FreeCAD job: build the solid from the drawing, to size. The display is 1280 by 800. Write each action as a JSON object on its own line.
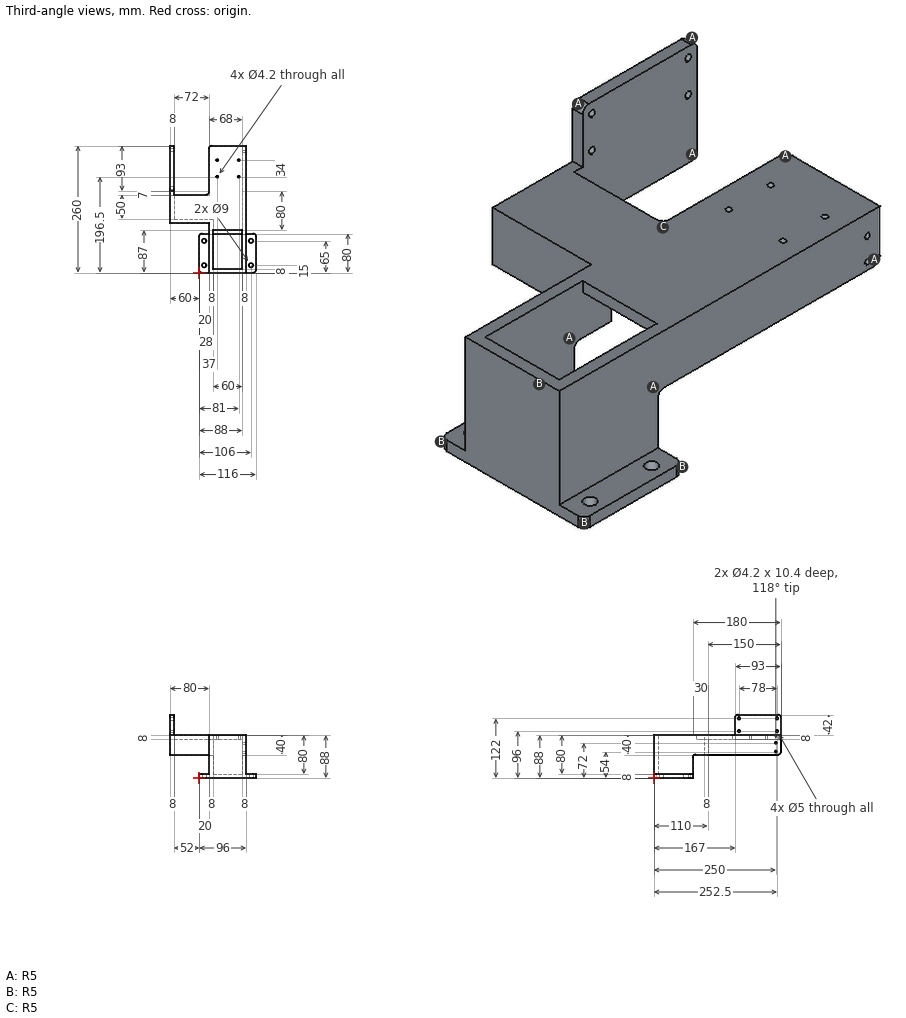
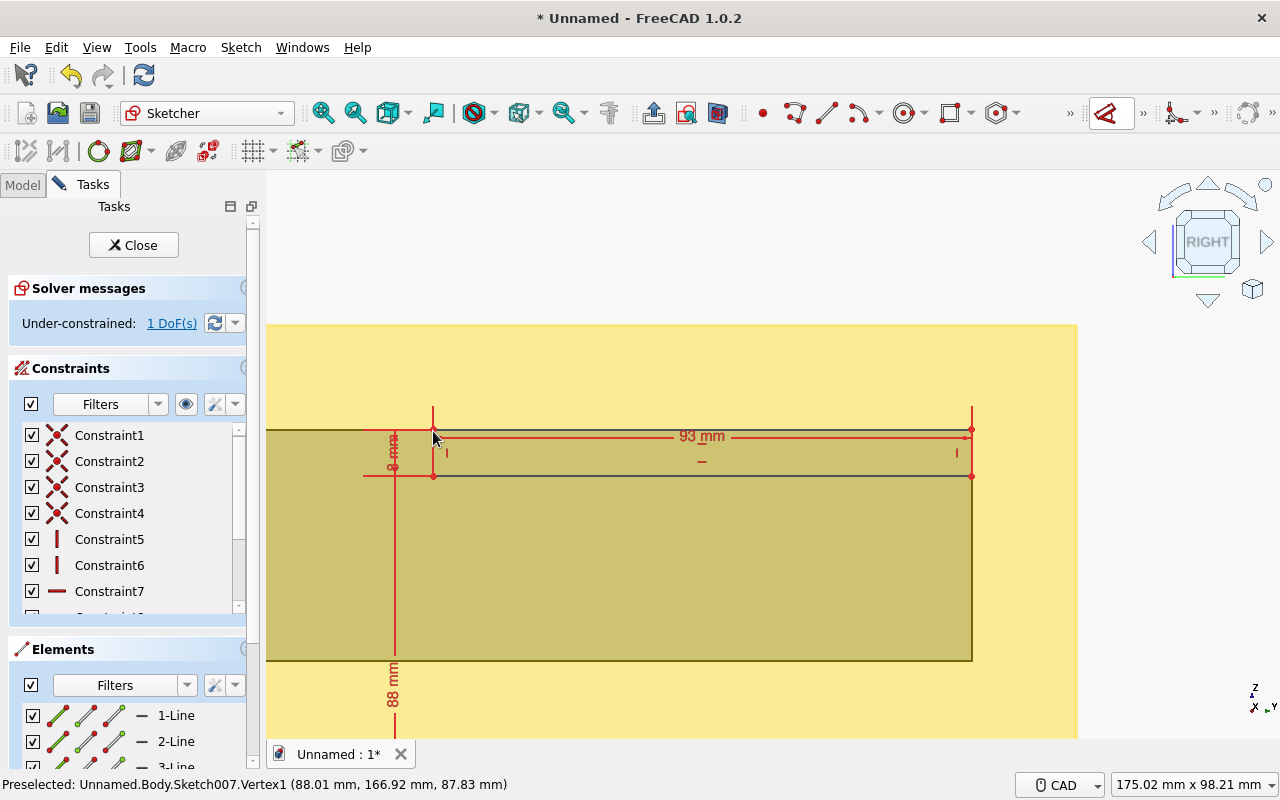
{"action": "left_click", "coordinate": [433, 430]}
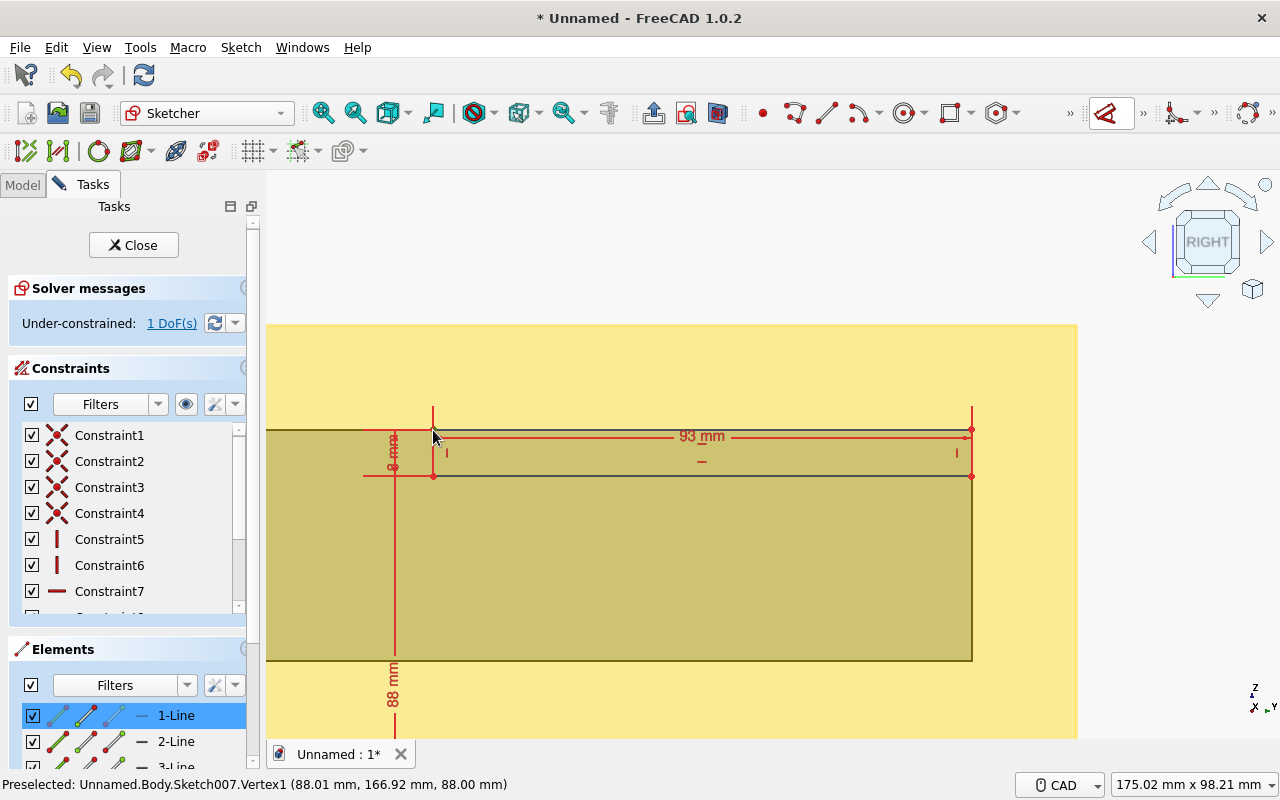
{"action": "key", "text": "l"}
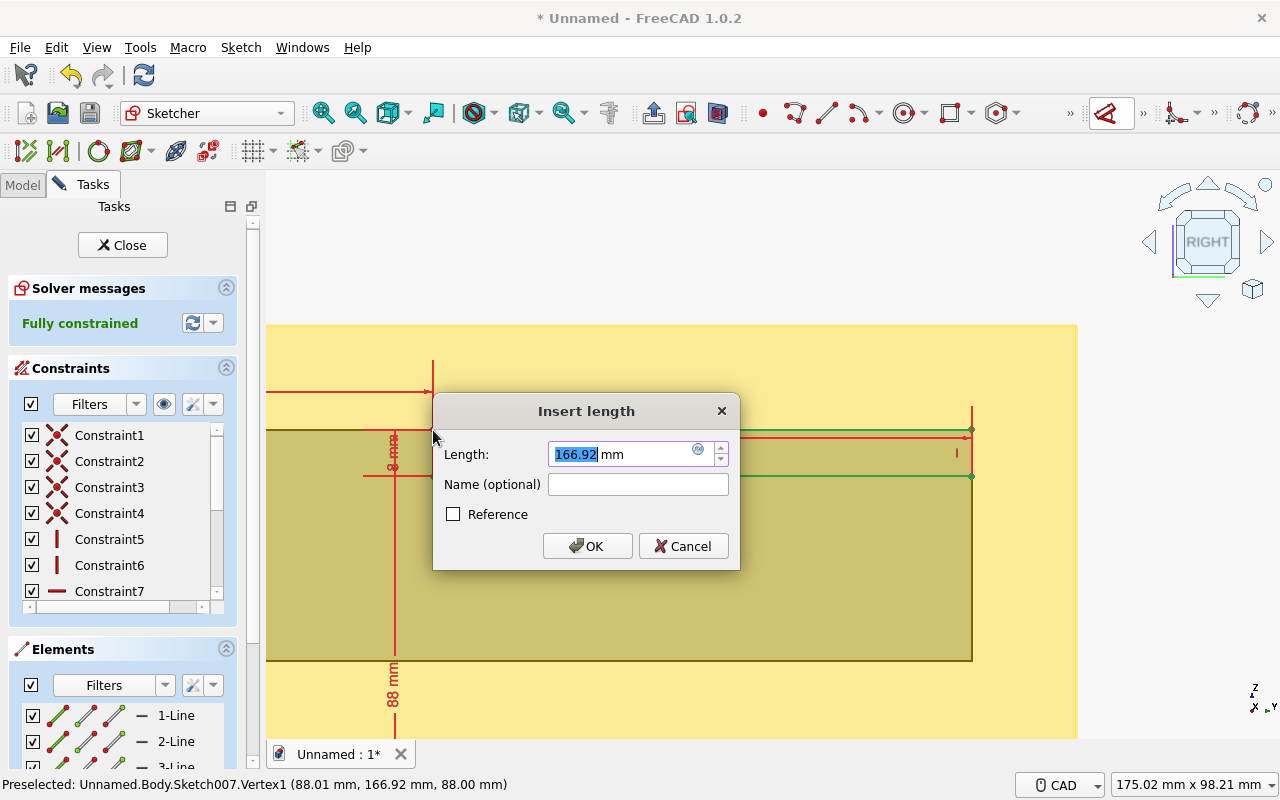
{"action": "type", "text": "167"}
{"action": "key", "text": "Return"}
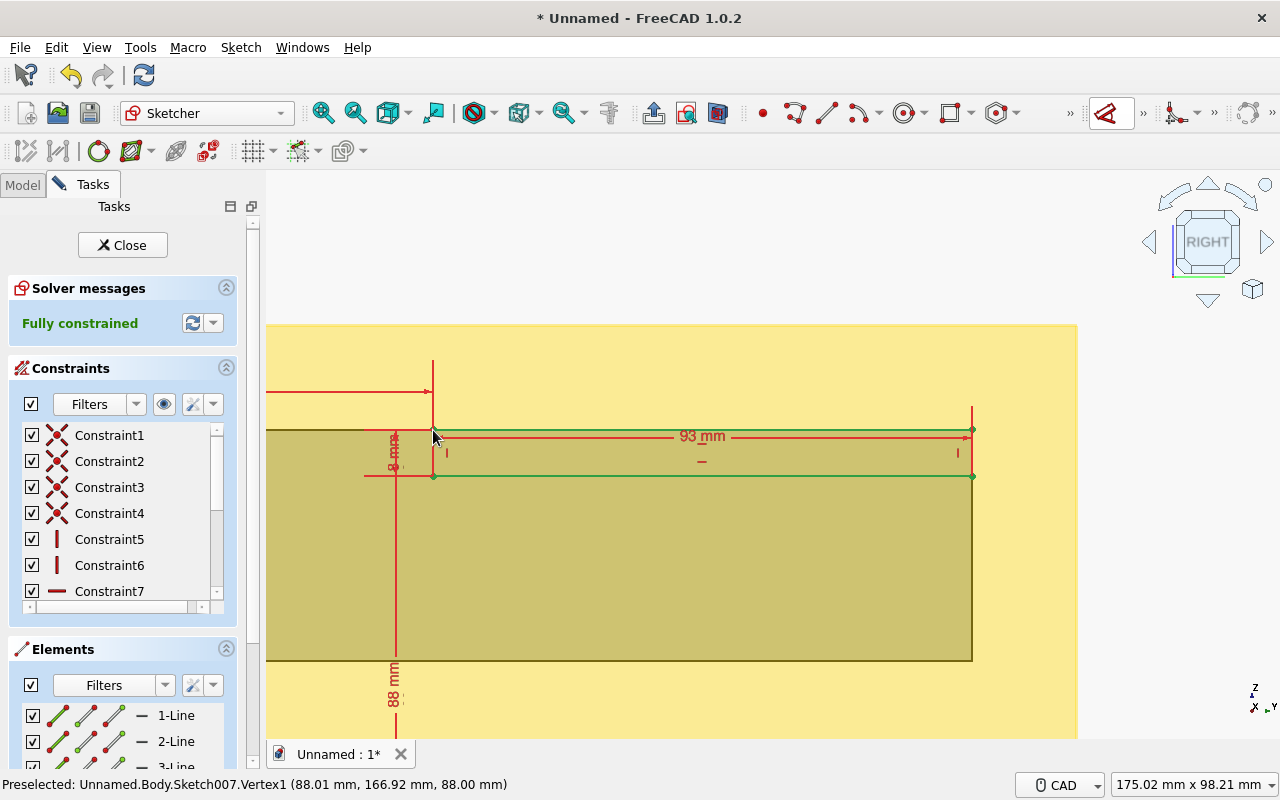
{"action": "left_click", "coordinate": [123, 245]}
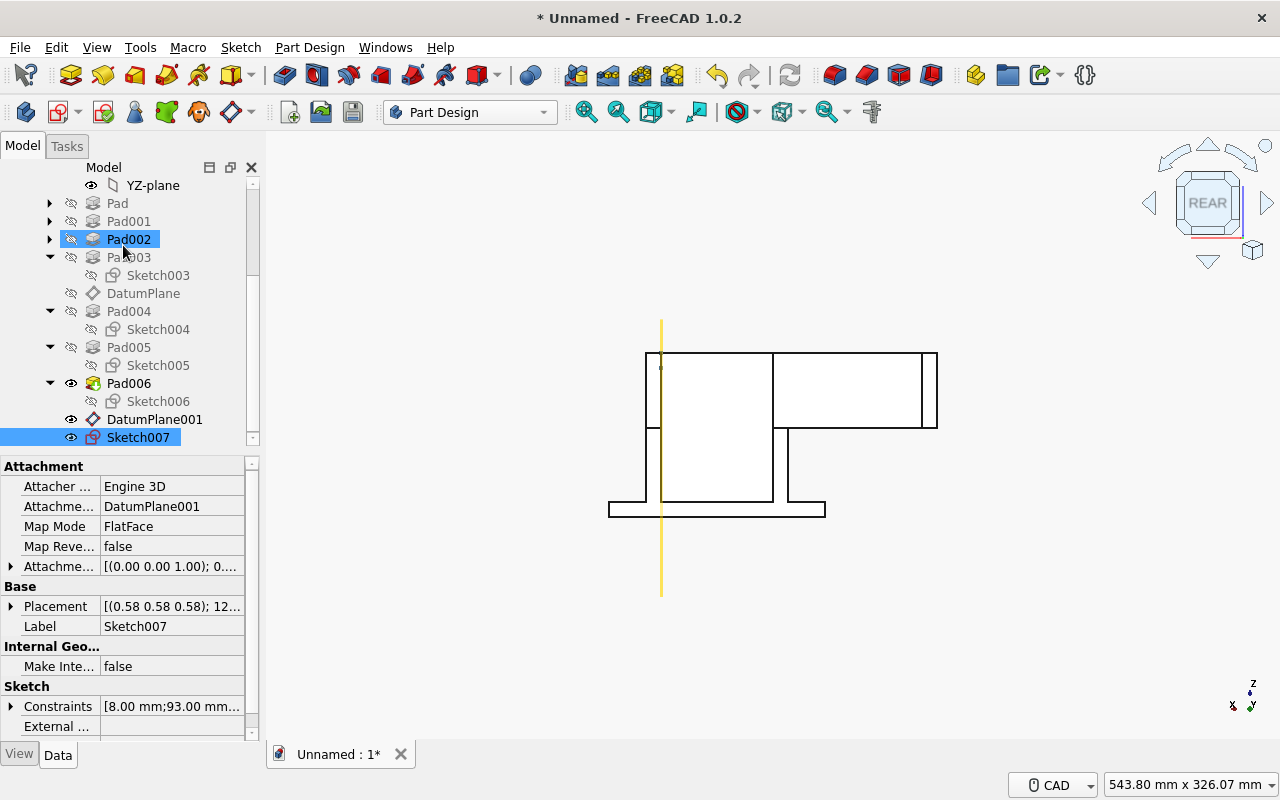
{"action": "left_click", "coordinate": [72, 76]}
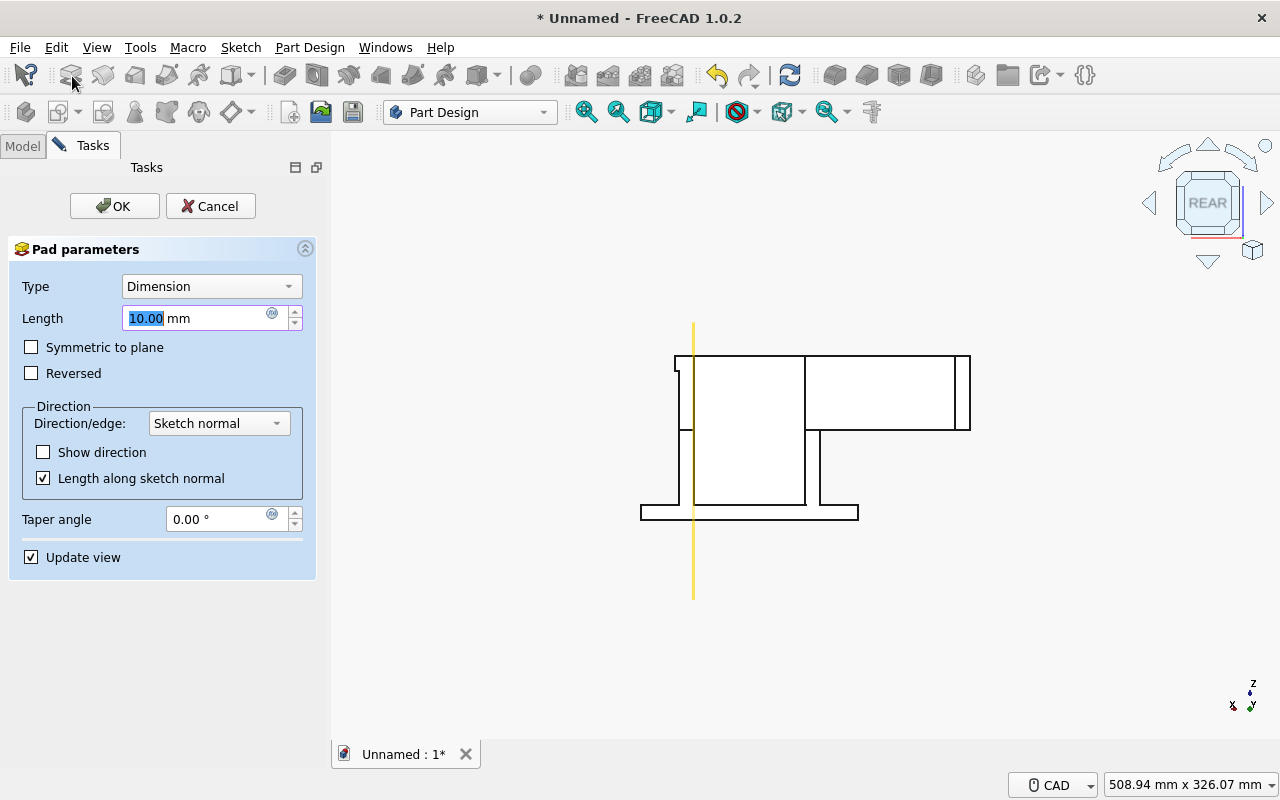
{"action": "type", "text": "68"}
{"action": "key", "text": "Tab"}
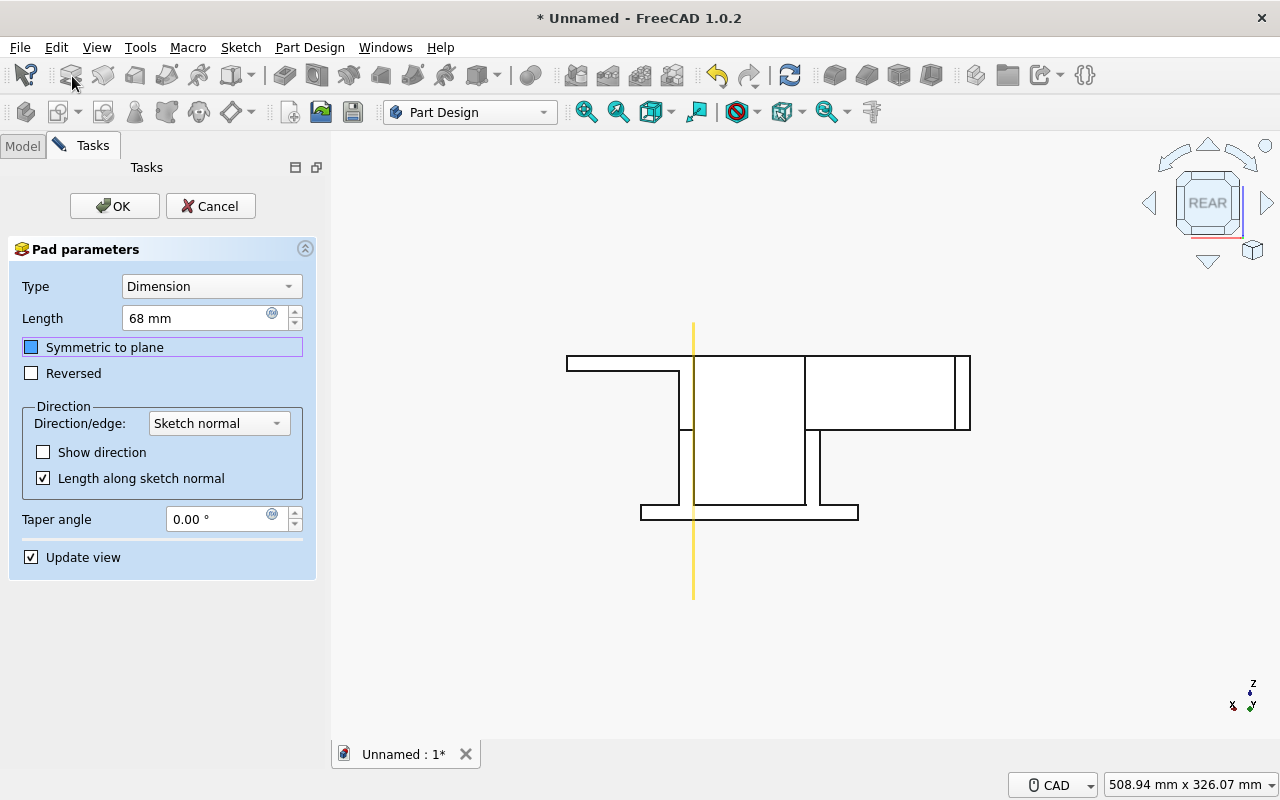
{"action": "left_click", "coordinate": [30, 373]}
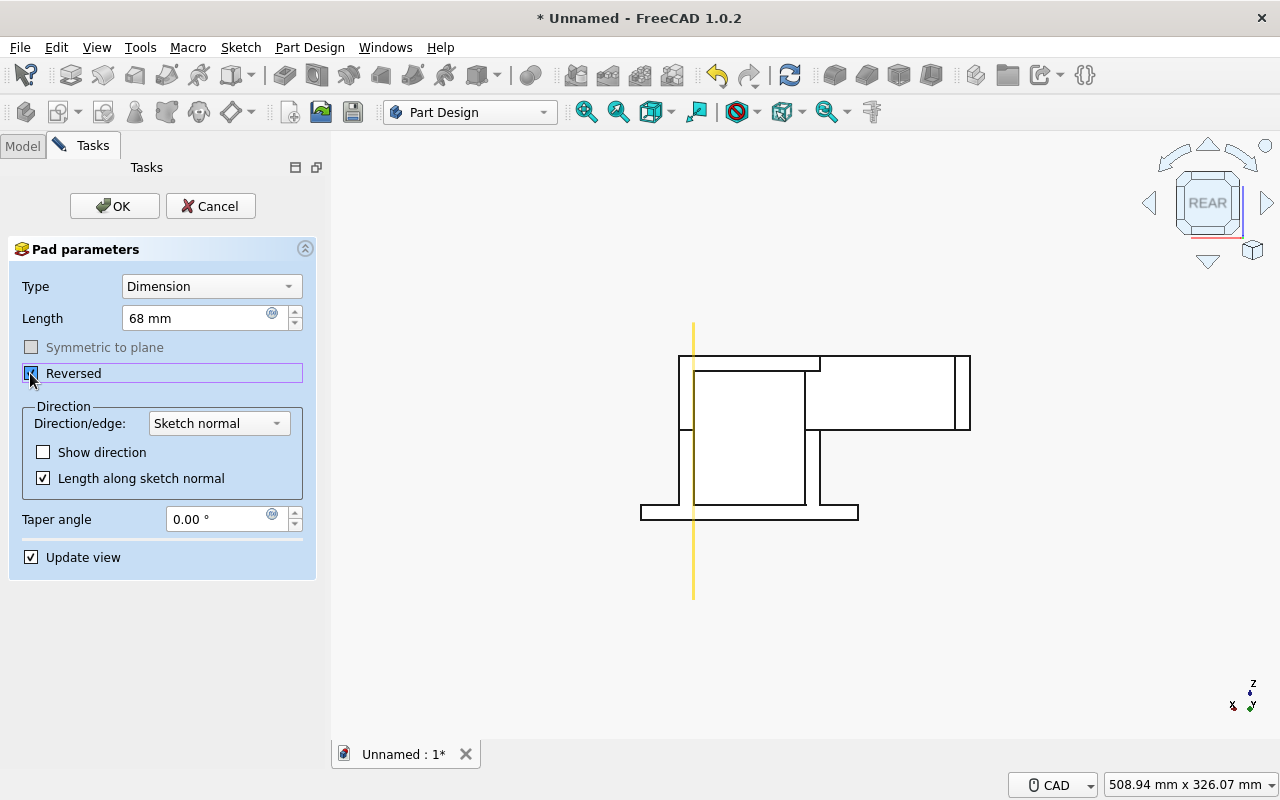
{"action": "left_click", "coordinate": [115, 206]}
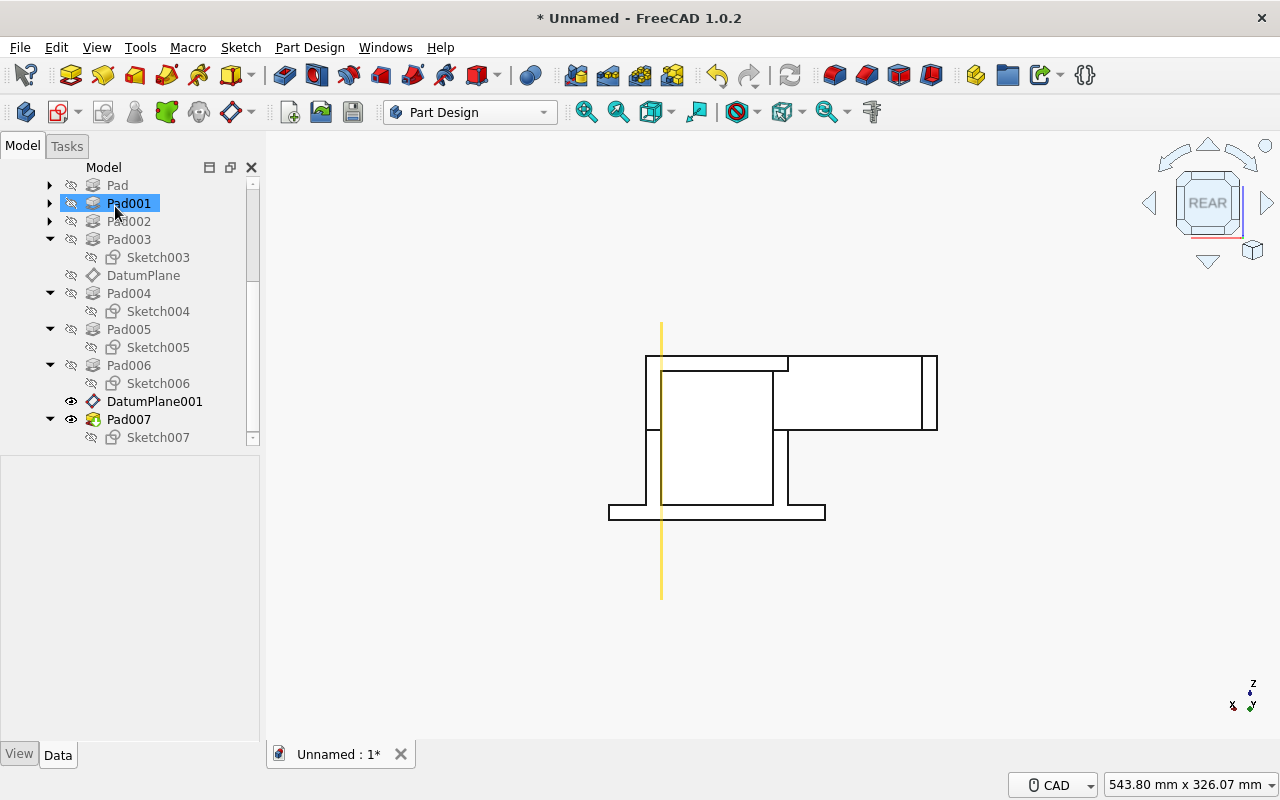
{"action": "left_click", "coordinate": [116, 401]}
{"action": "key", "text": "space"}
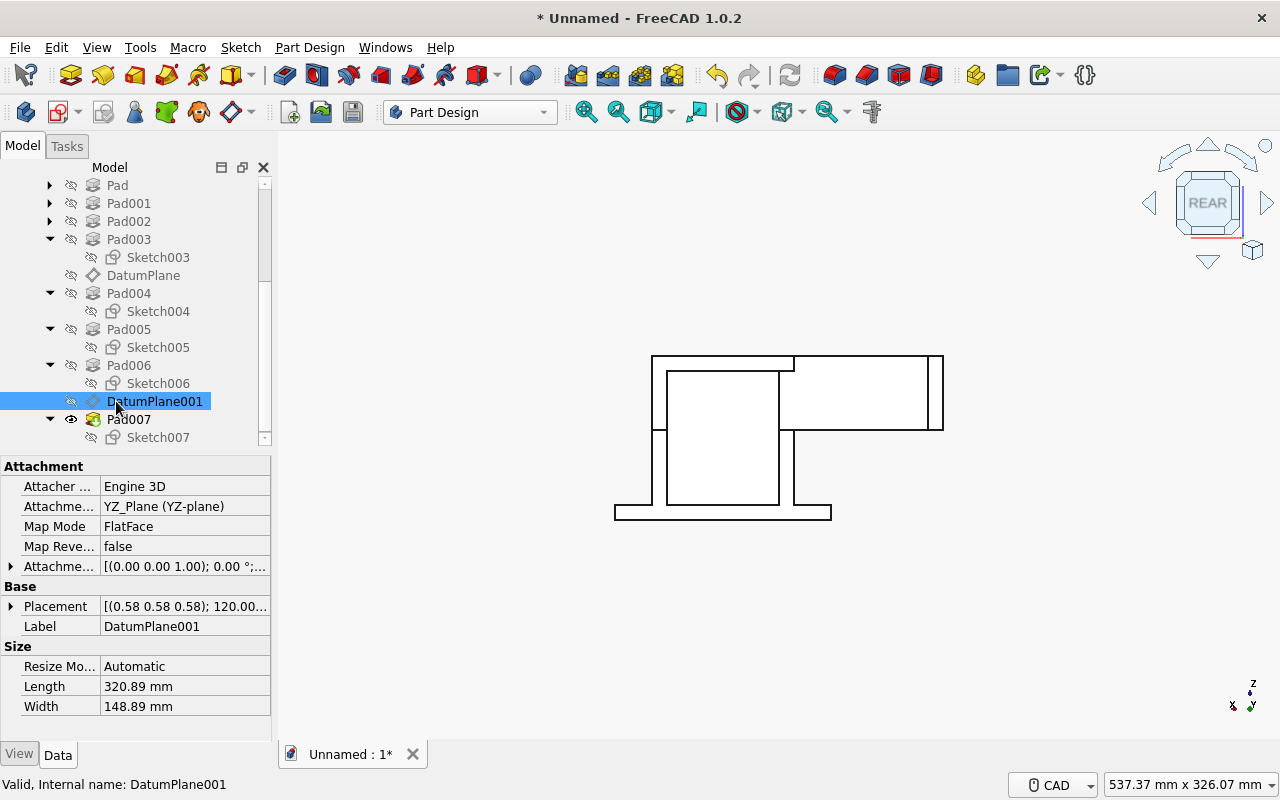
{"action": "left_click", "coordinate": [588, 112]}